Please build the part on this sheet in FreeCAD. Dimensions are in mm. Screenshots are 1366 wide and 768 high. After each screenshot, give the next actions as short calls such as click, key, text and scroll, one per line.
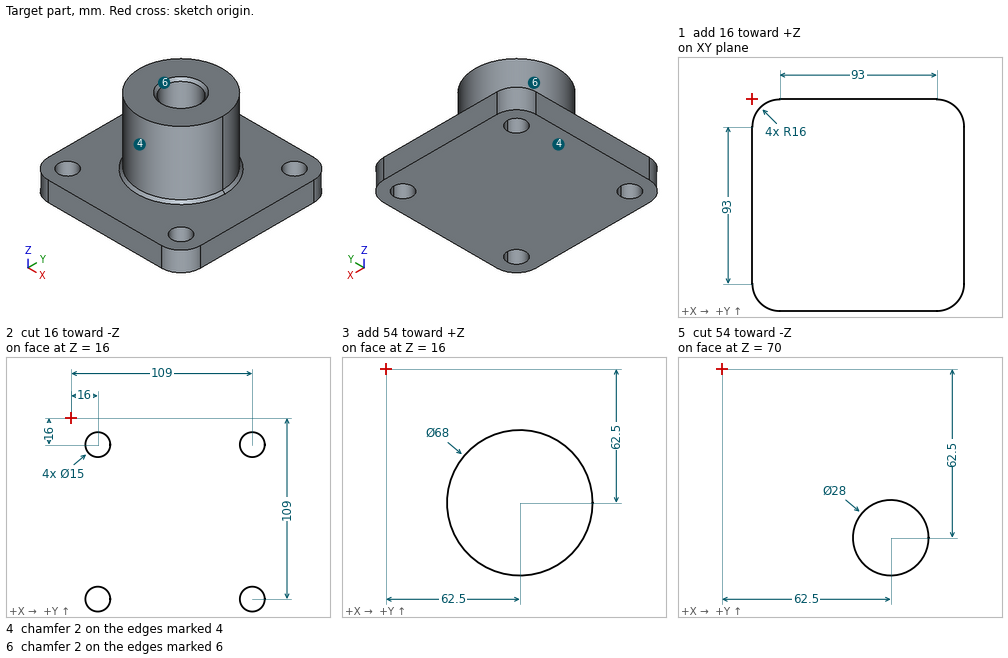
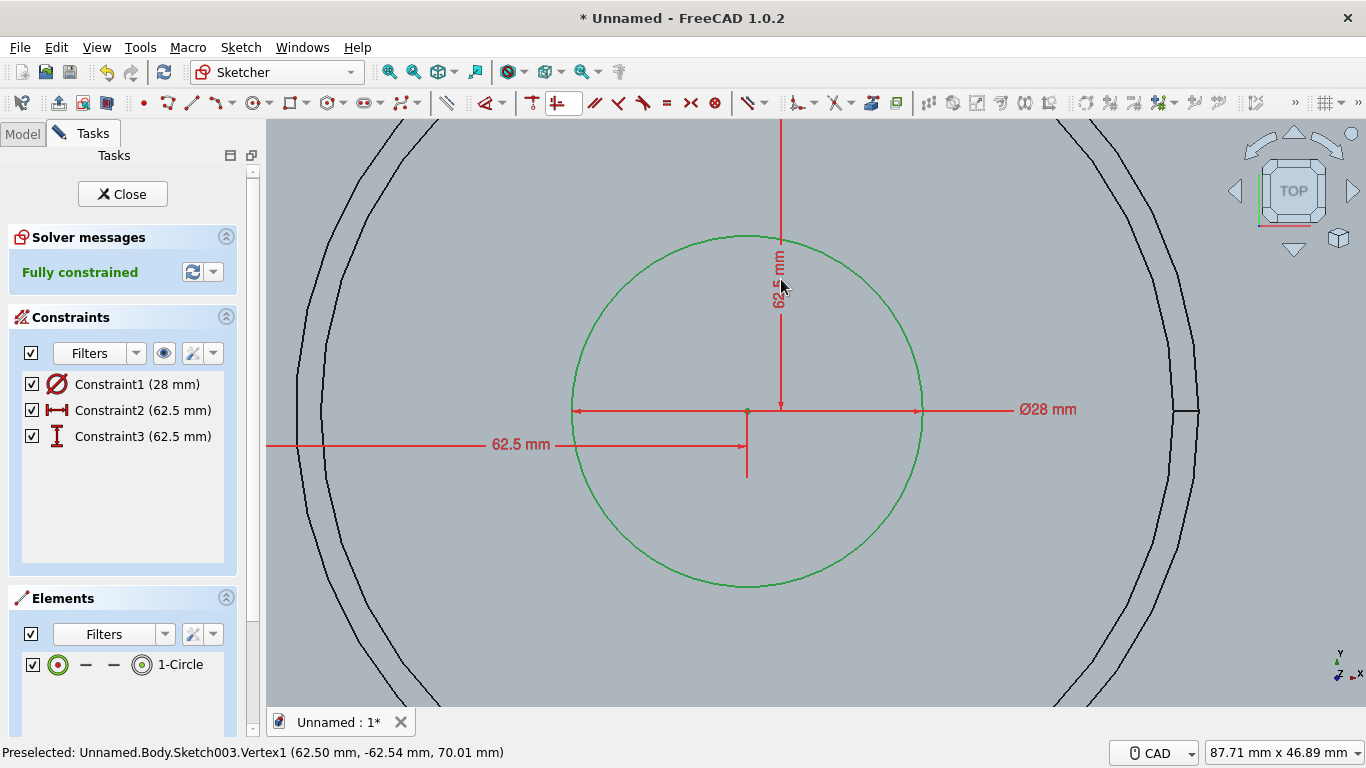
click(123, 194)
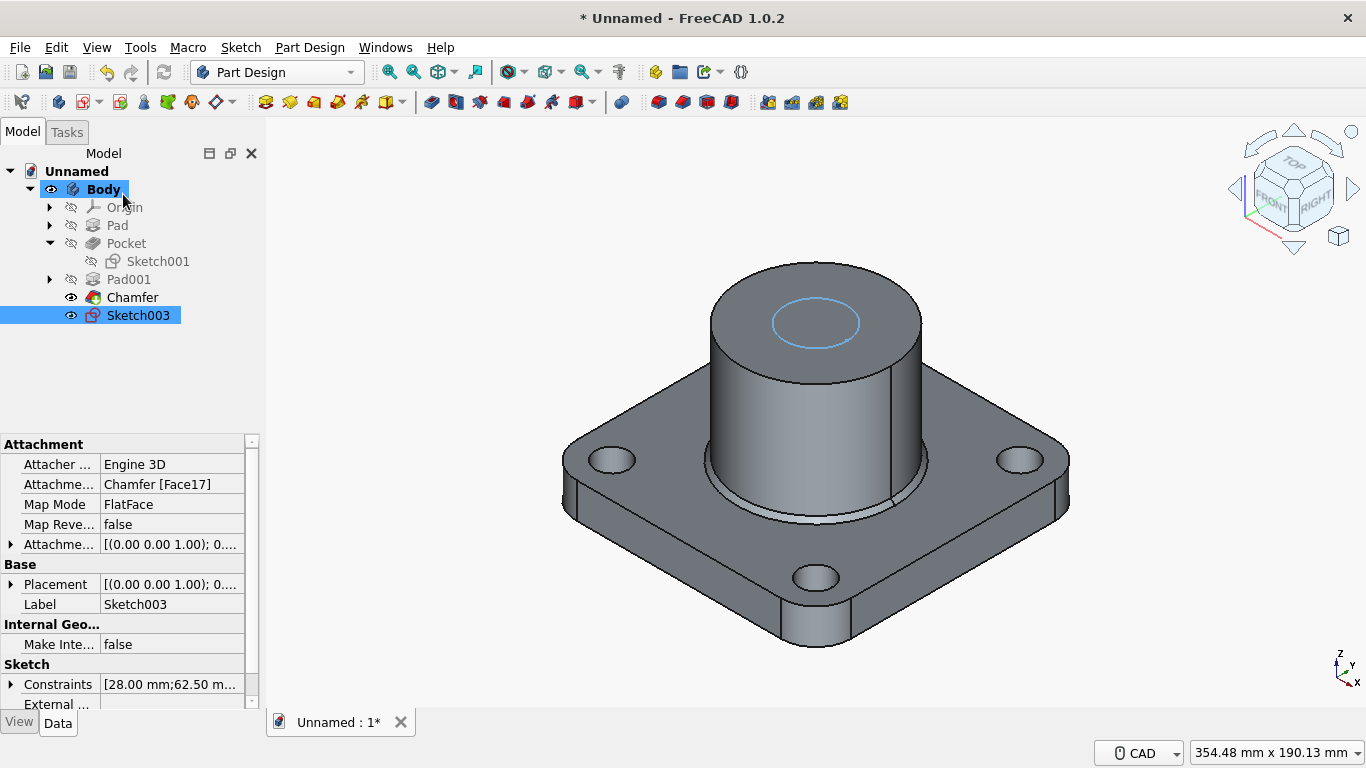
click(432, 102)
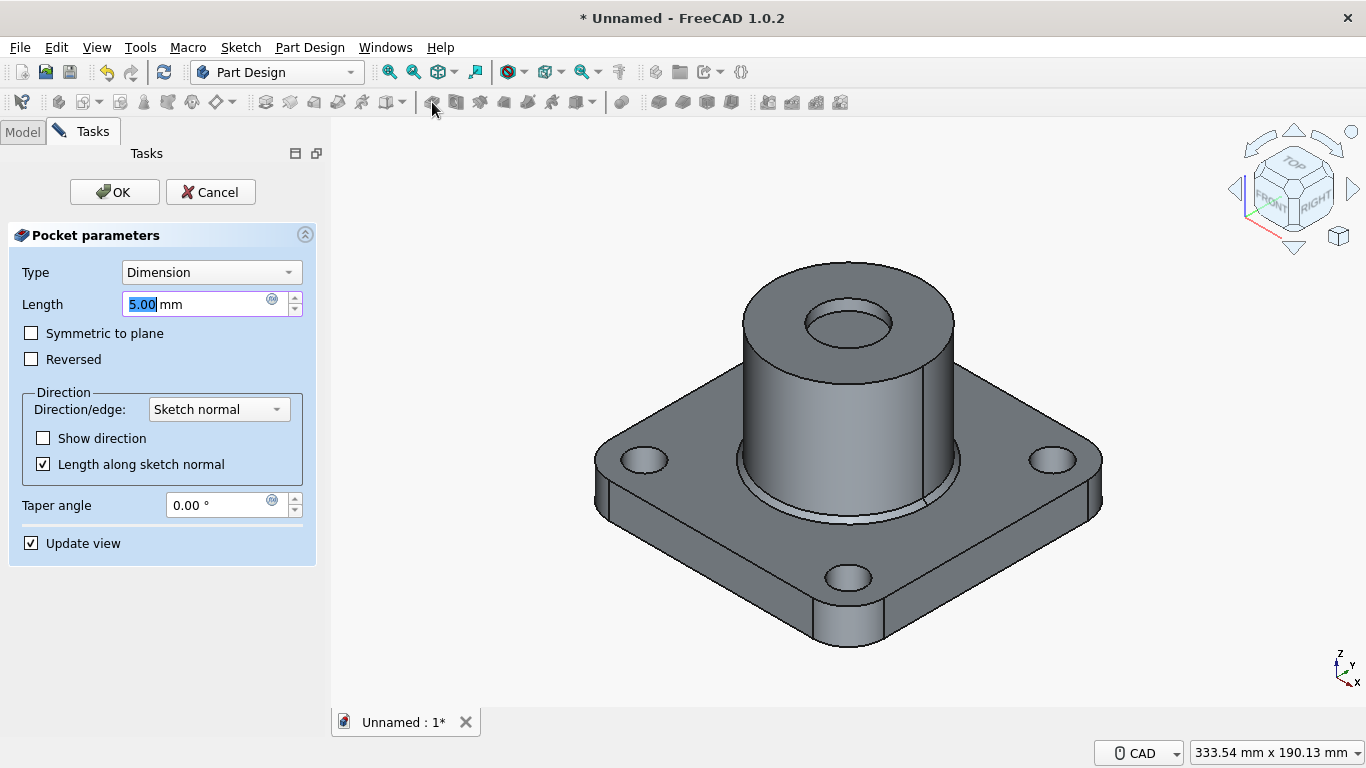
text(54)
key(Tab)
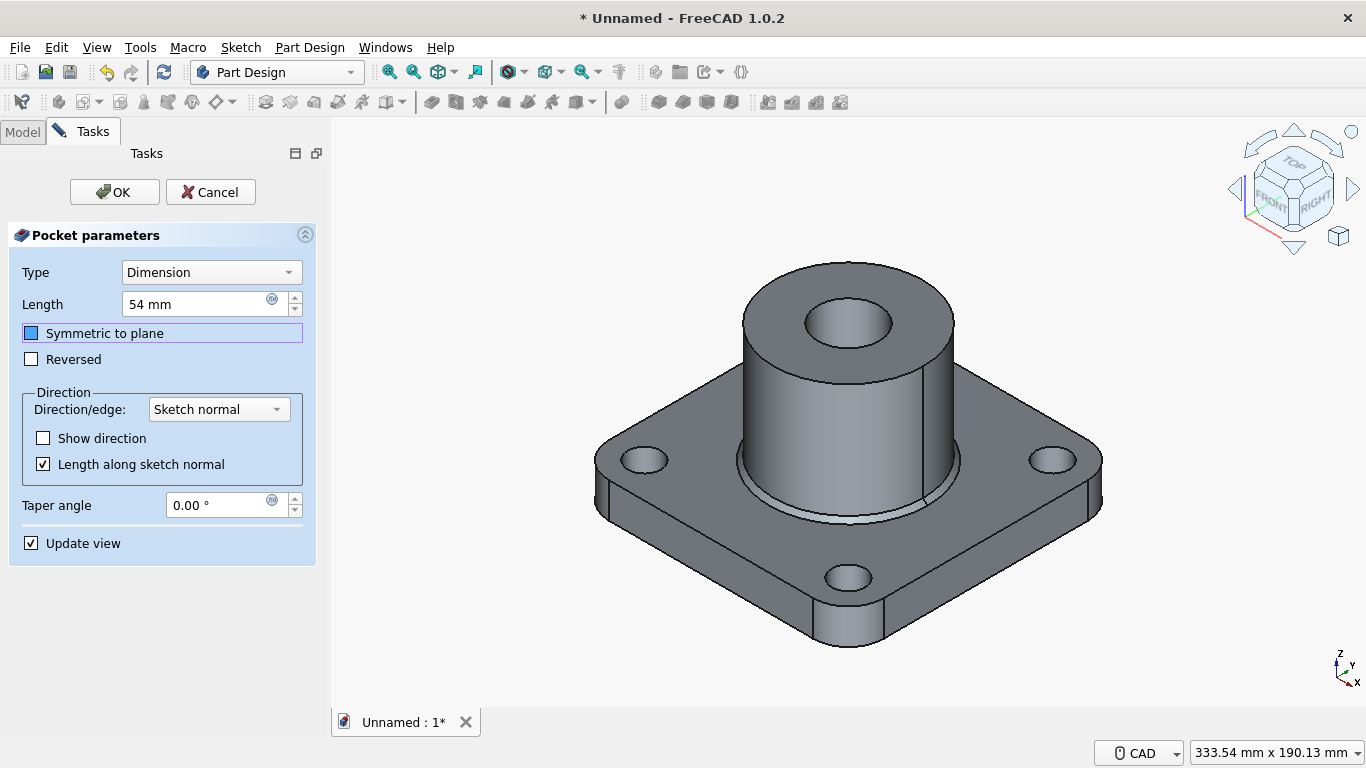
click(115, 192)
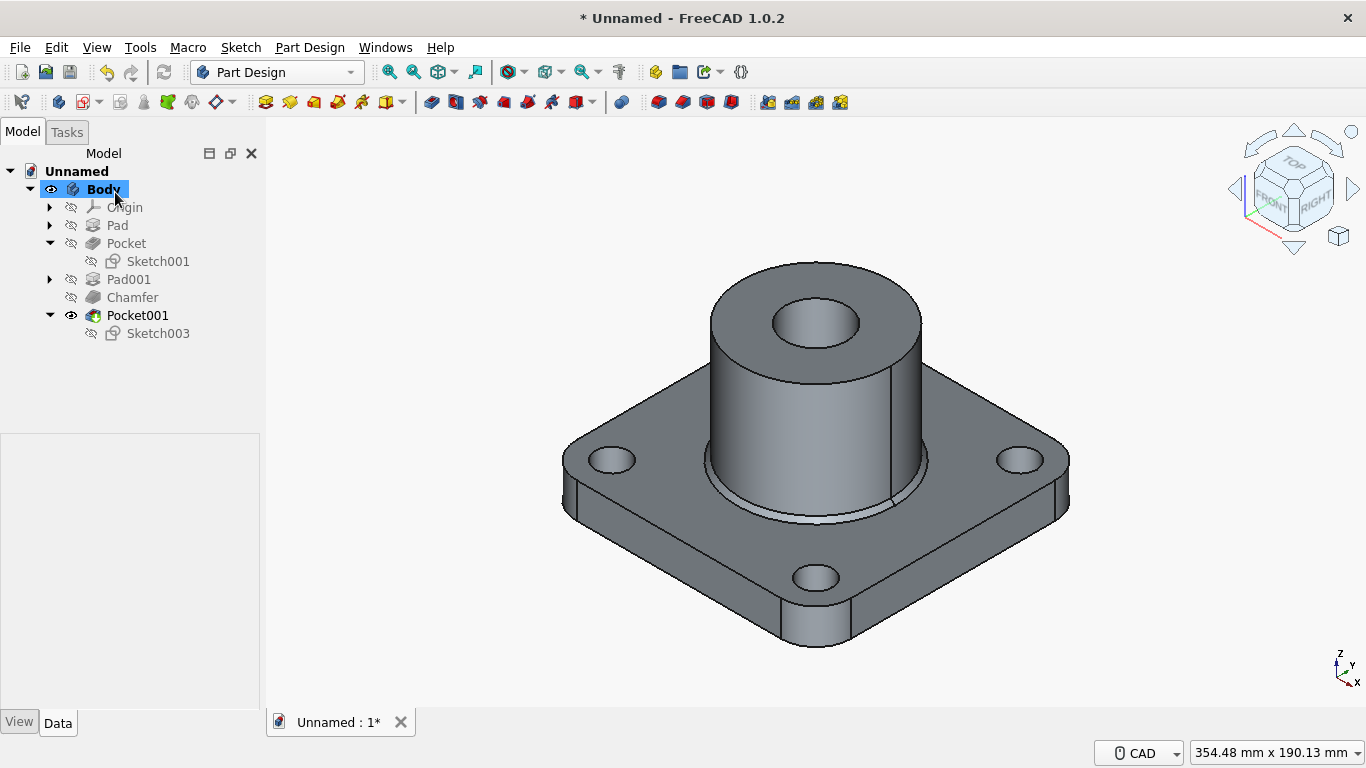
click(785, 305)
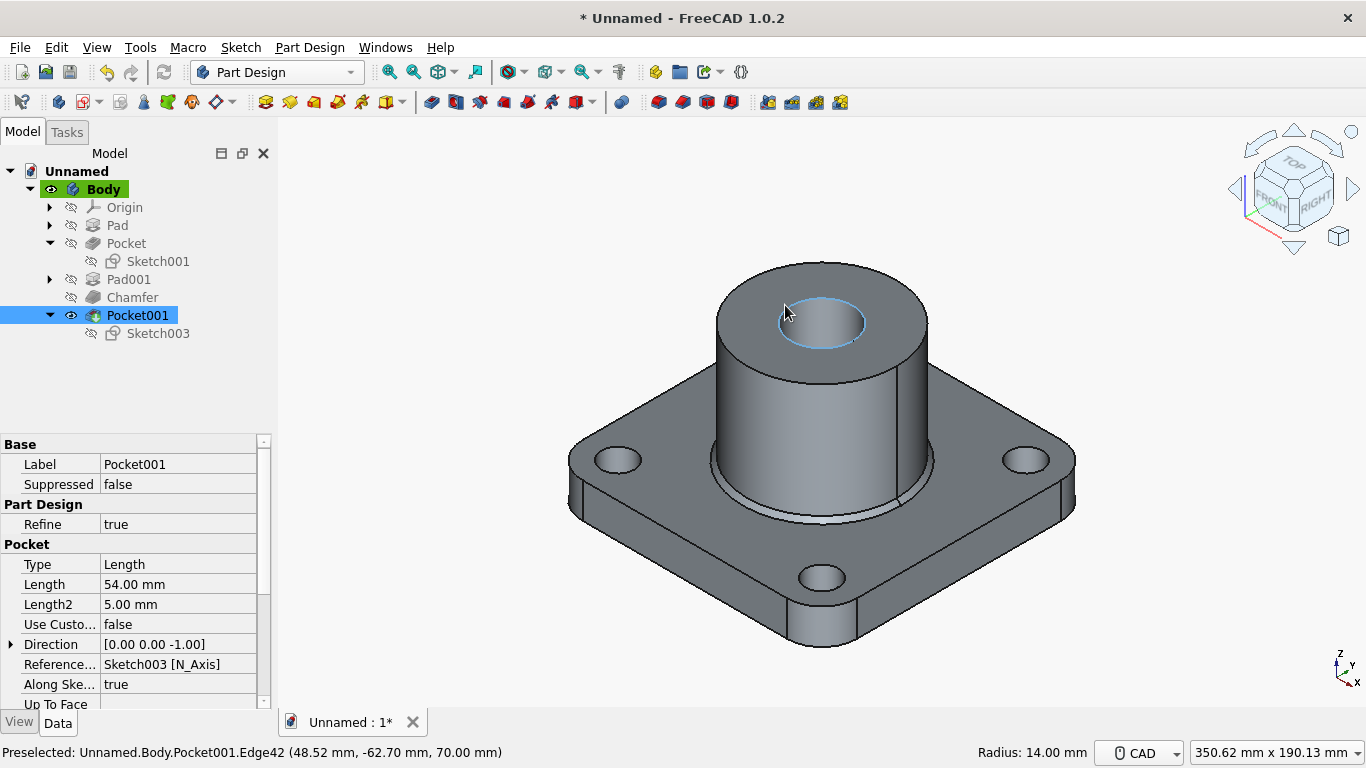
click(684, 102)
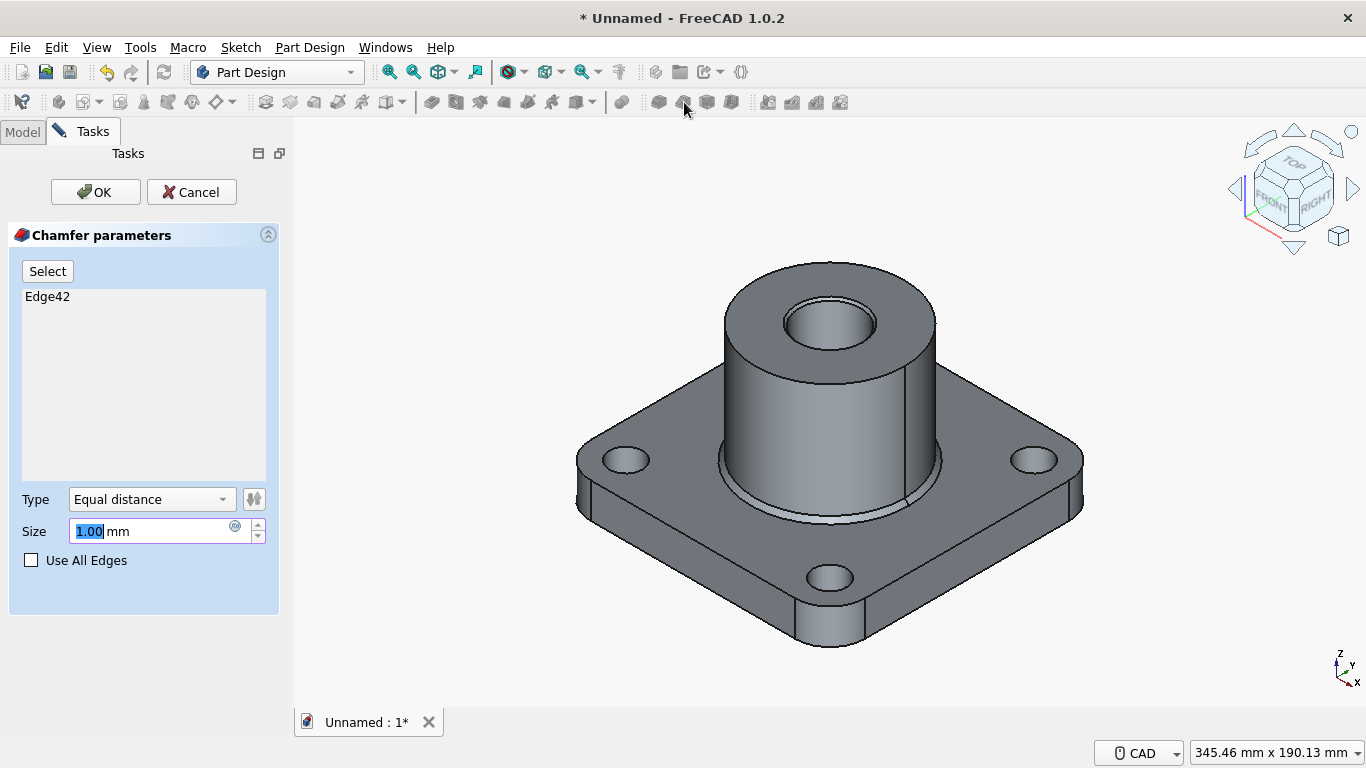
text(2)
key(Tab)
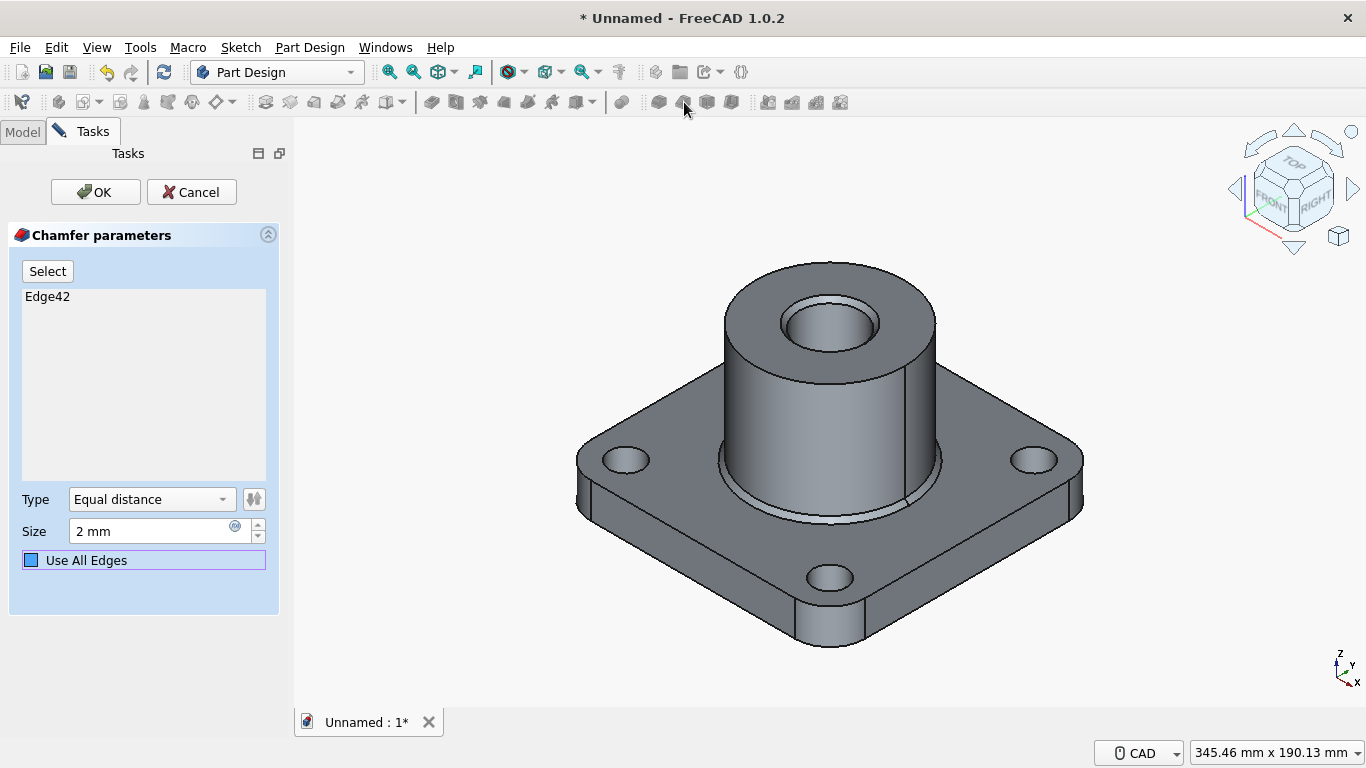
click(96, 192)